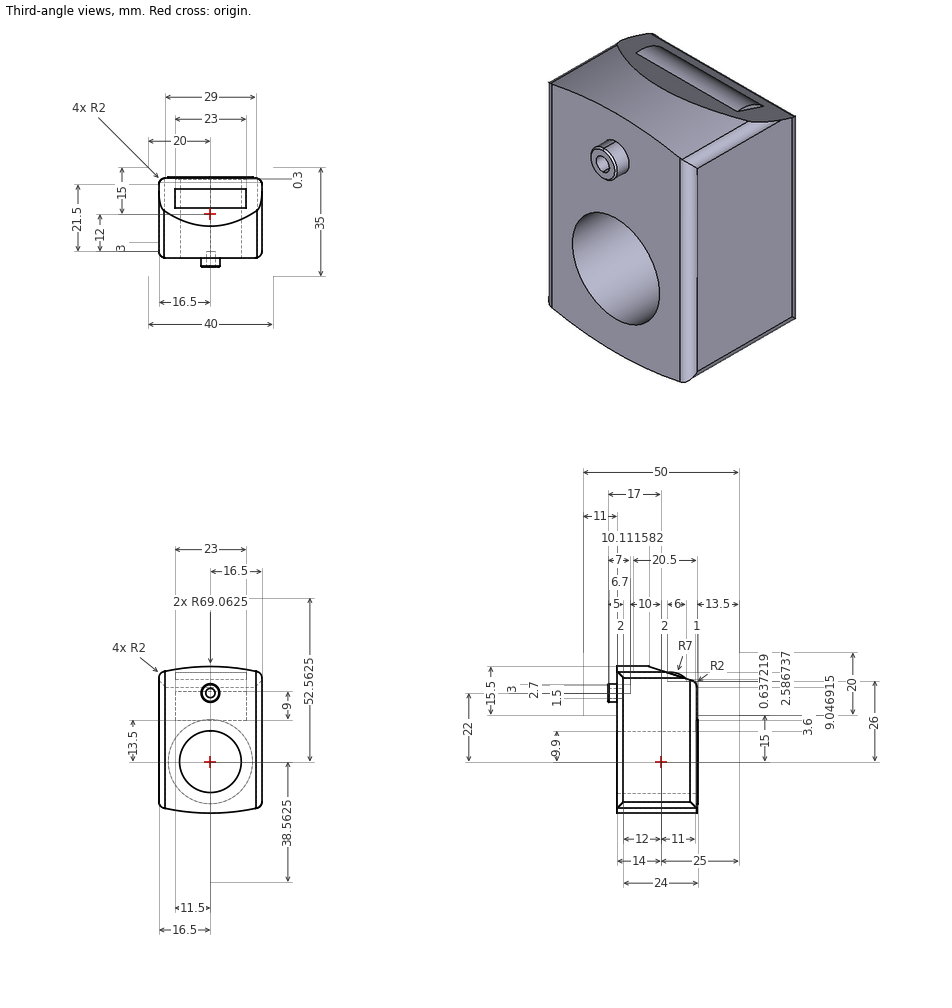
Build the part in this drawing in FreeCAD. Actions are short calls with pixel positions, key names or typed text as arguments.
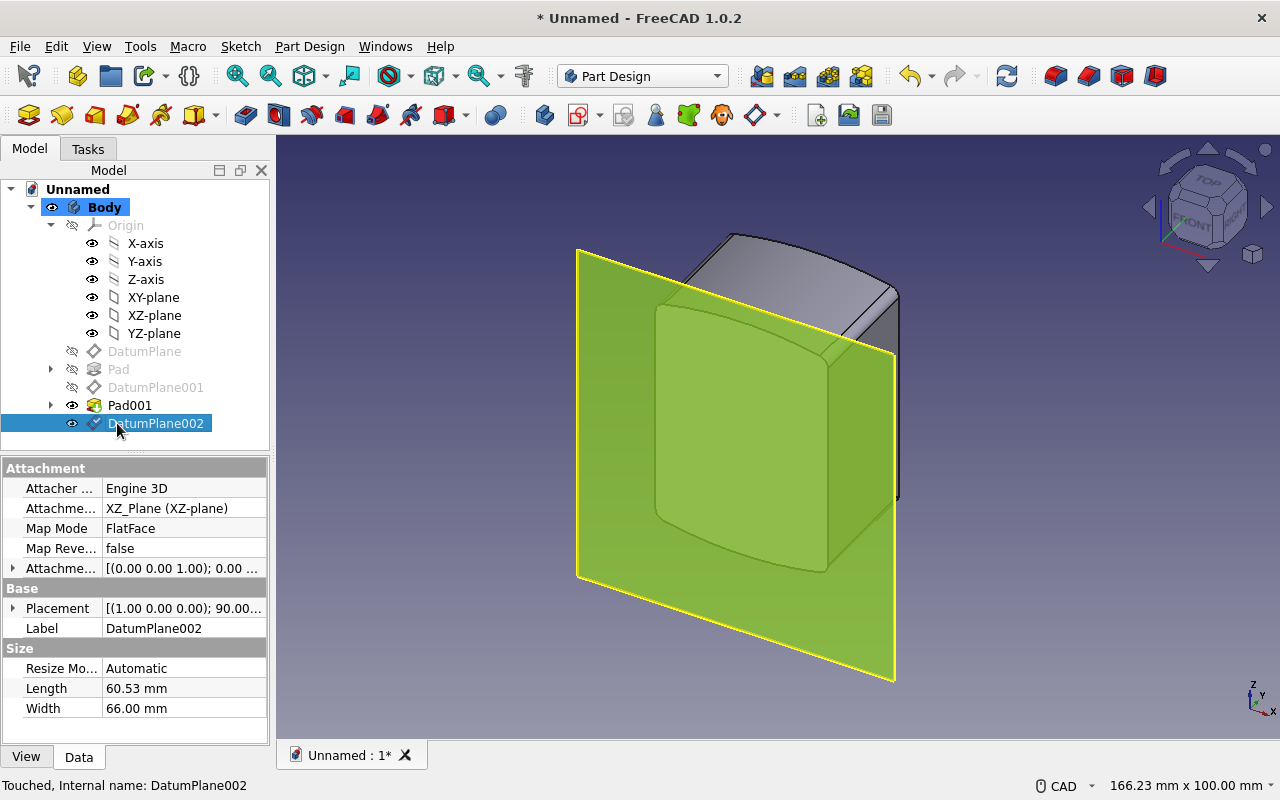
click(578, 116)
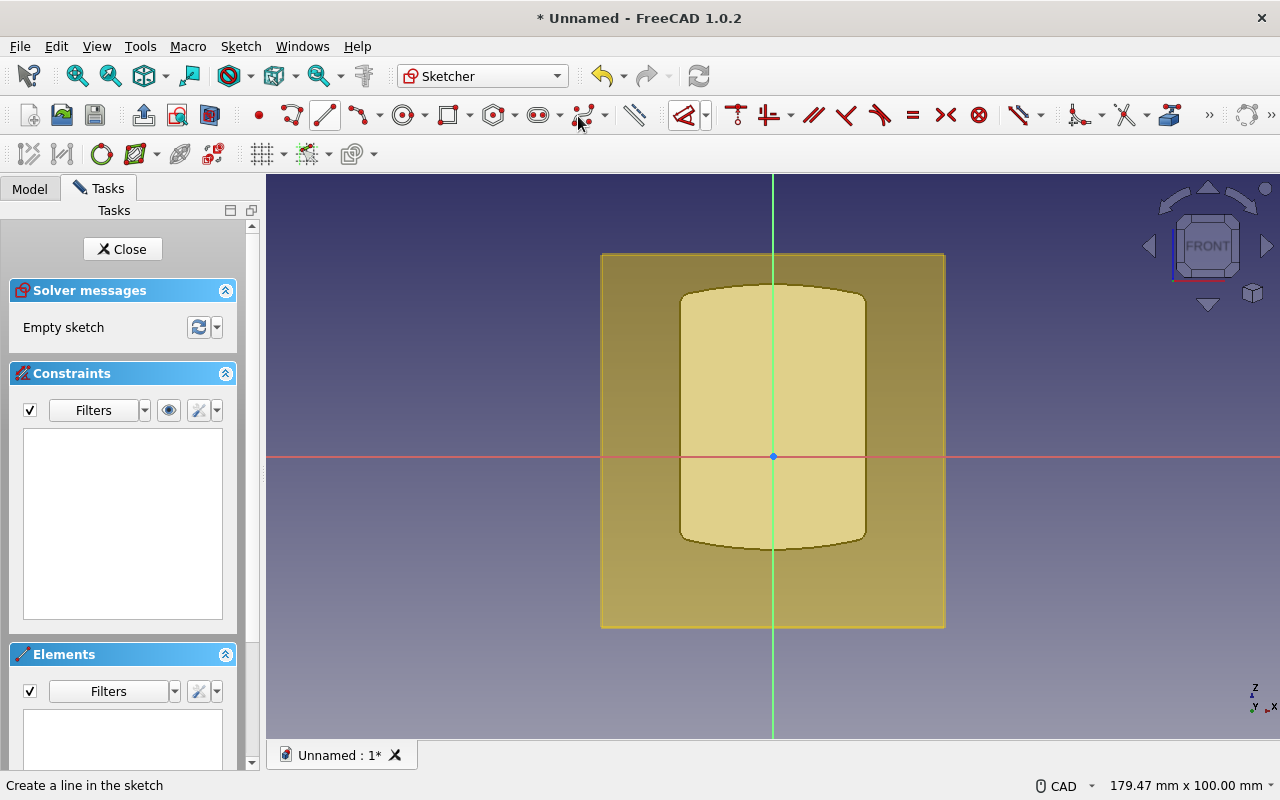
scroll(912, 337, up, 2)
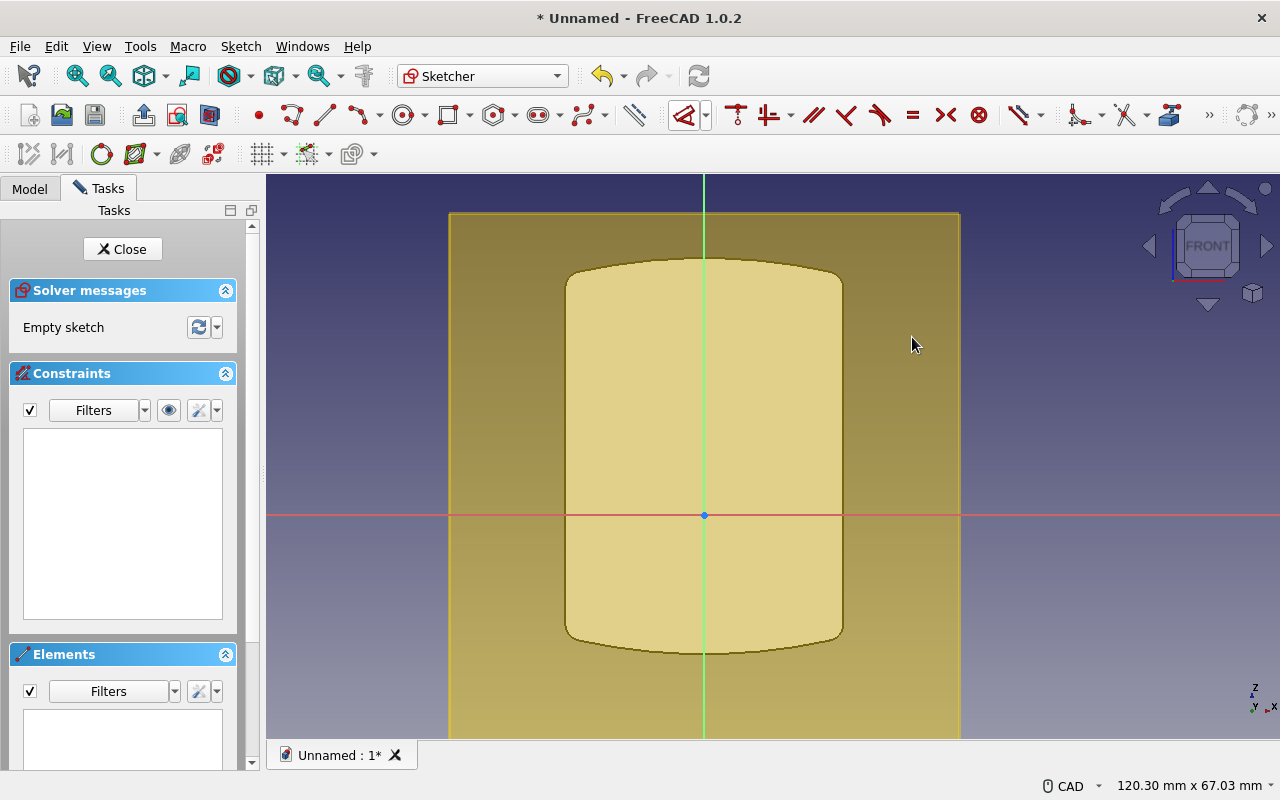
click(325, 116)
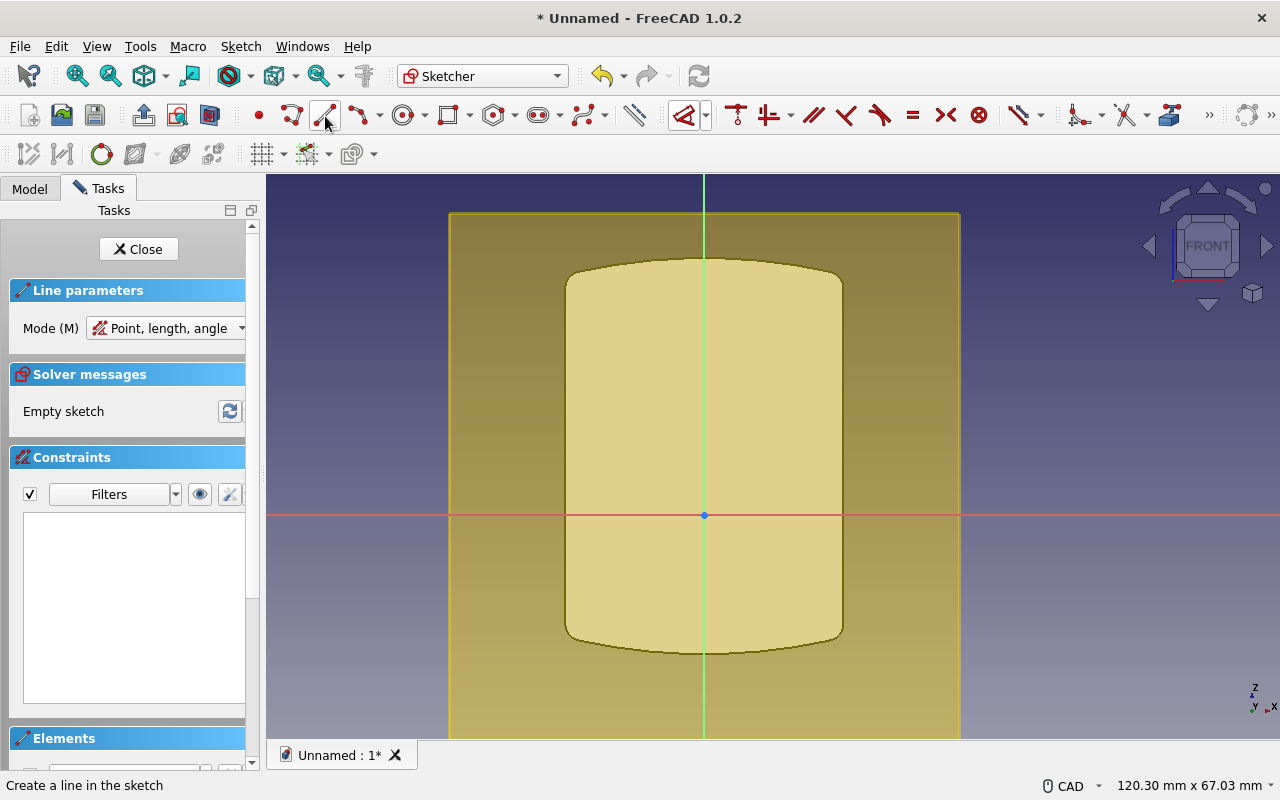
click(565, 624)
click(565, 288)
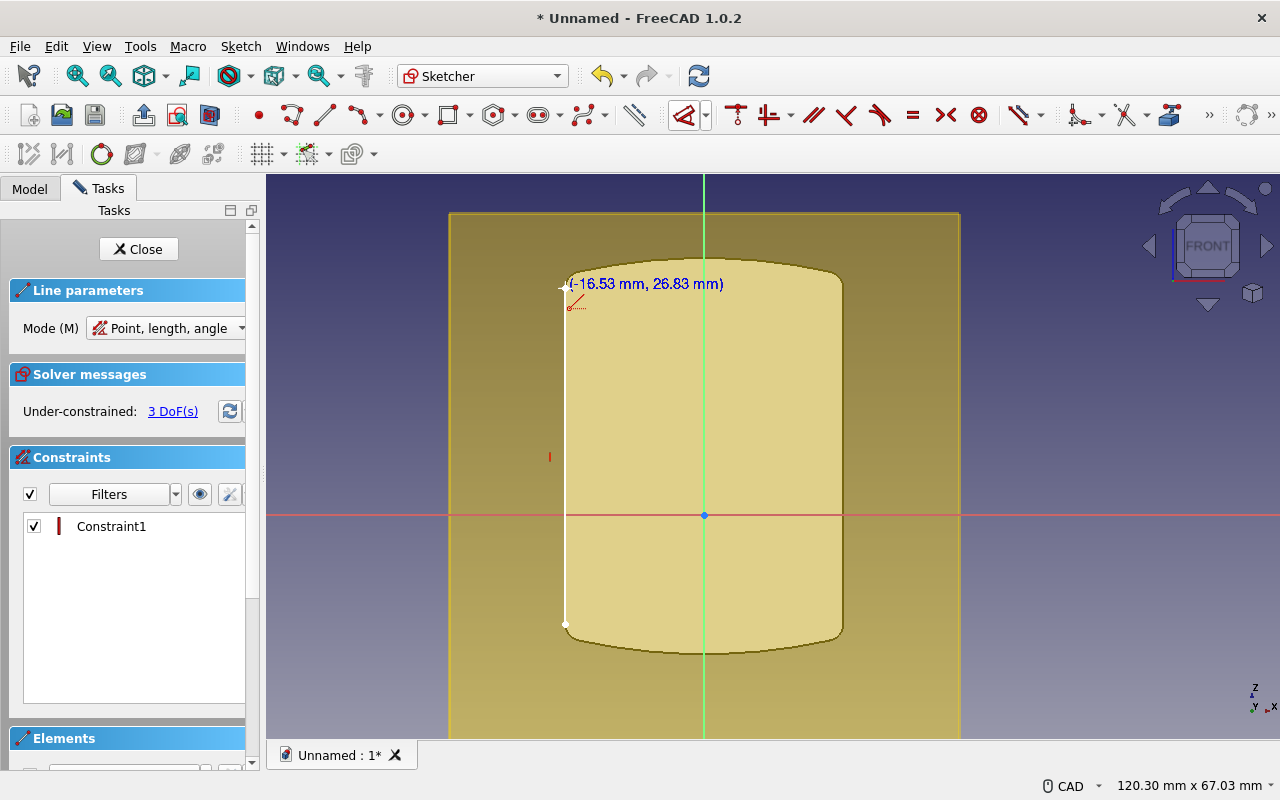
click(843, 288)
click(843, 624)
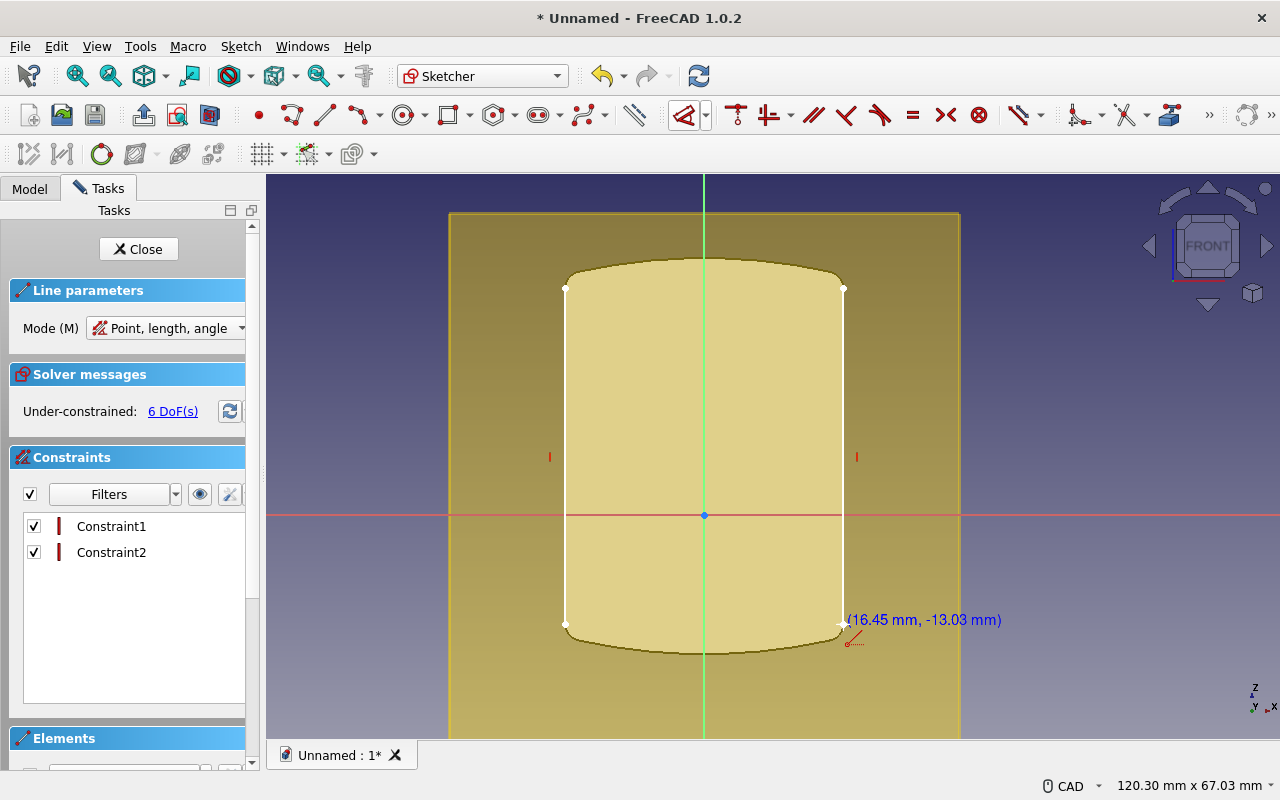
click(358, 116)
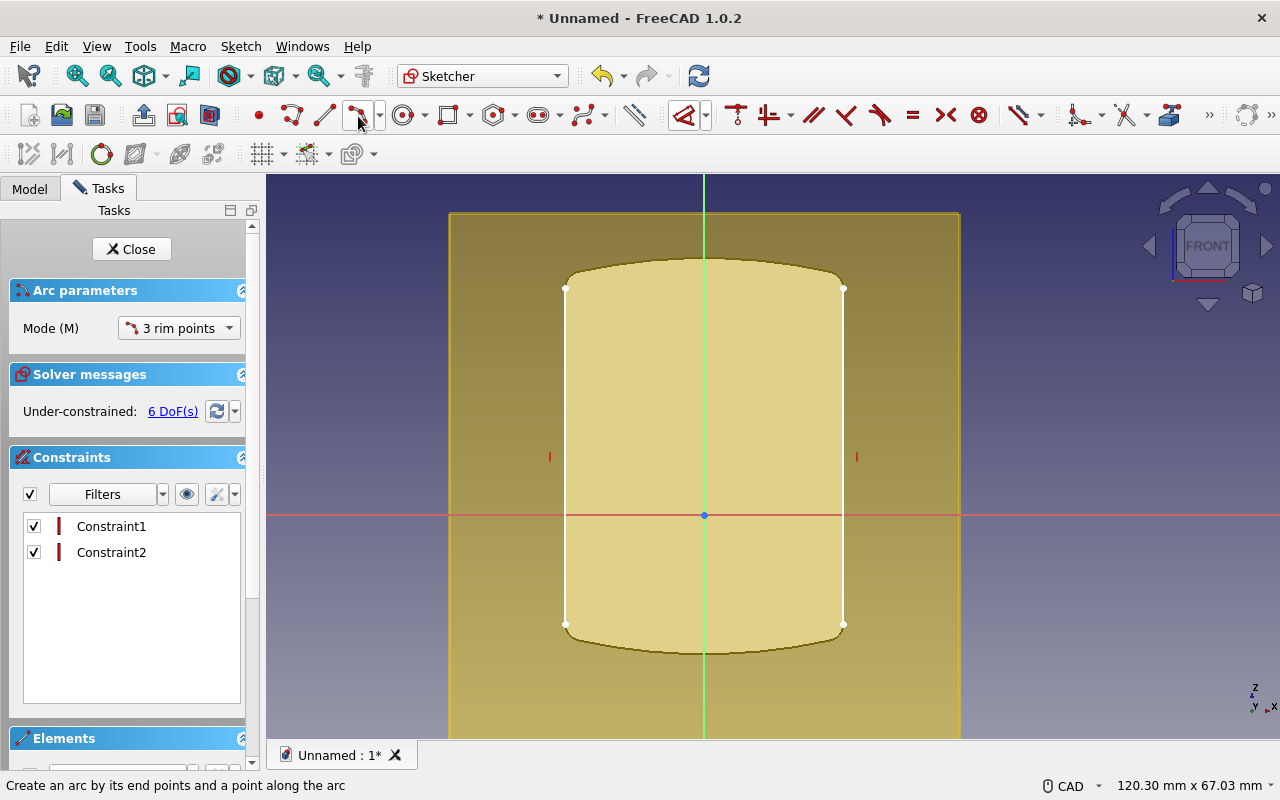
click(565, 289)
click(578, 272)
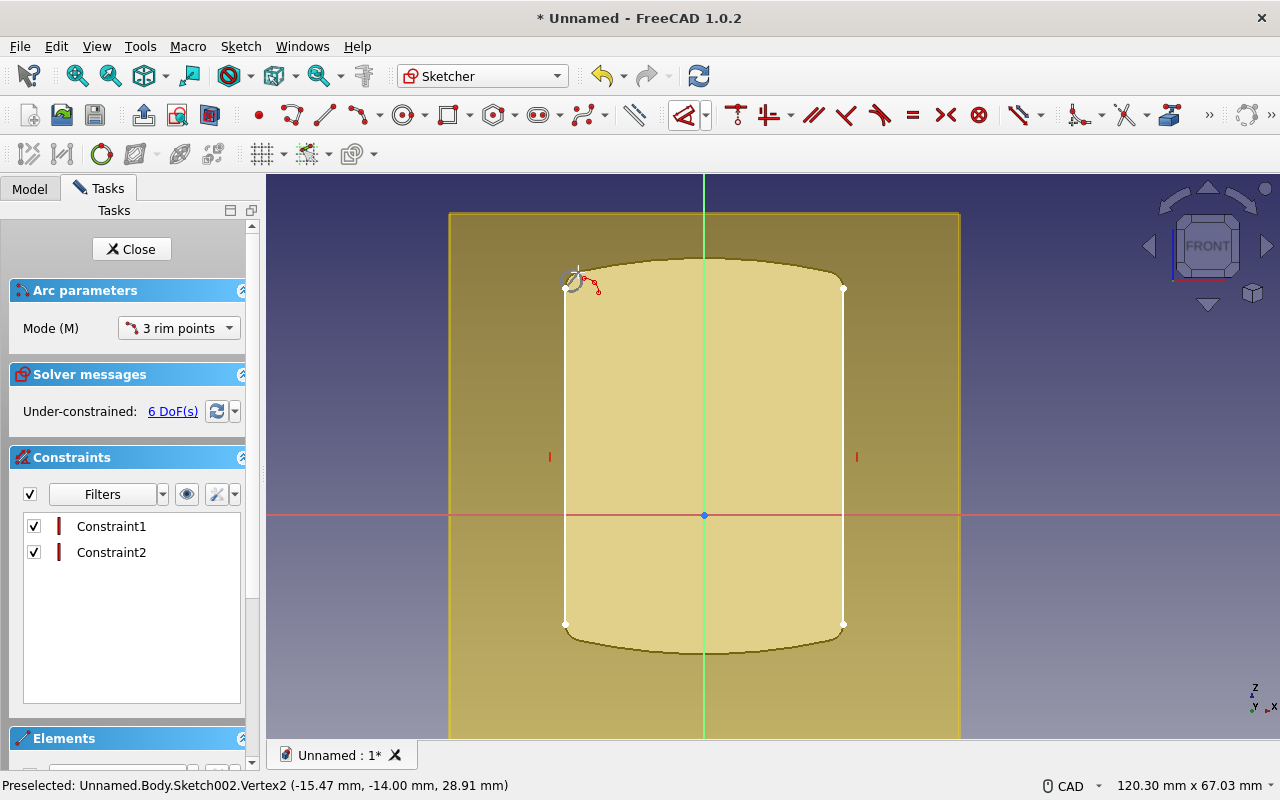
scroll(569, 278, up, 8)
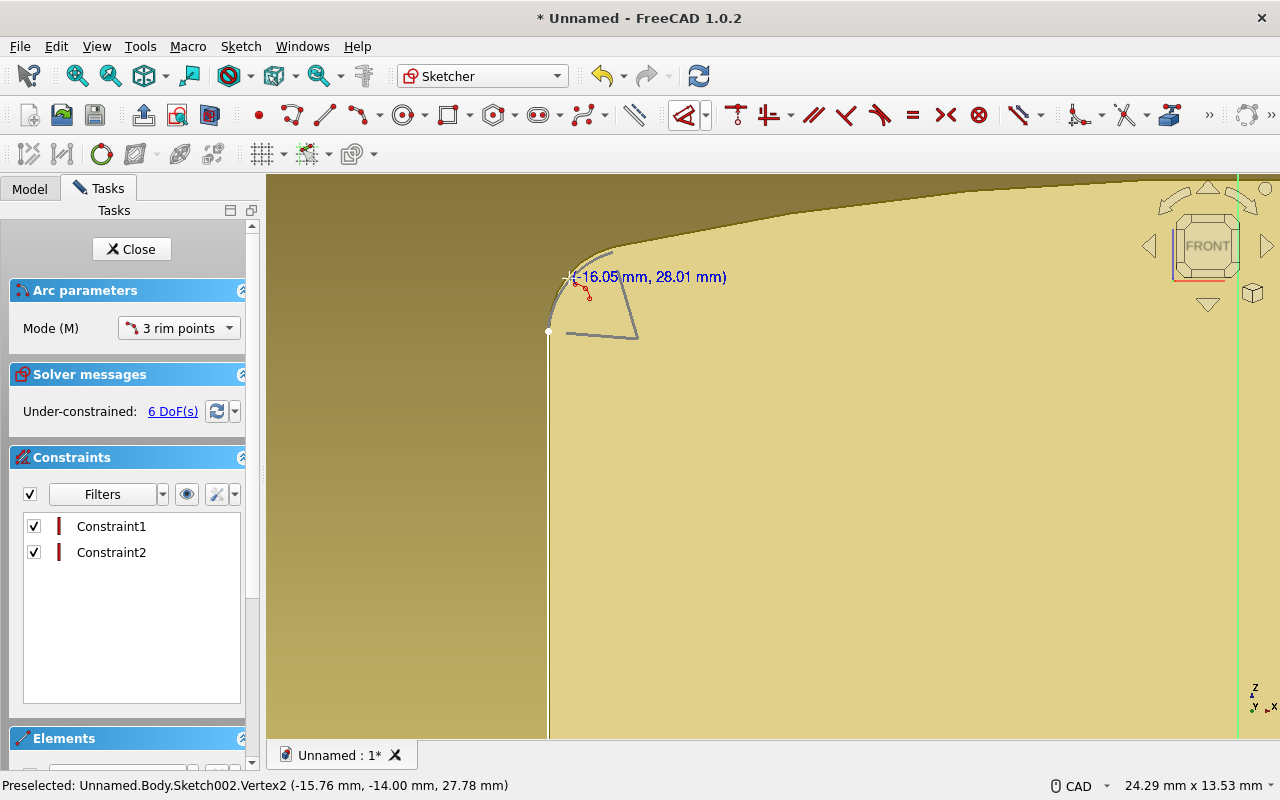
click(568, 276)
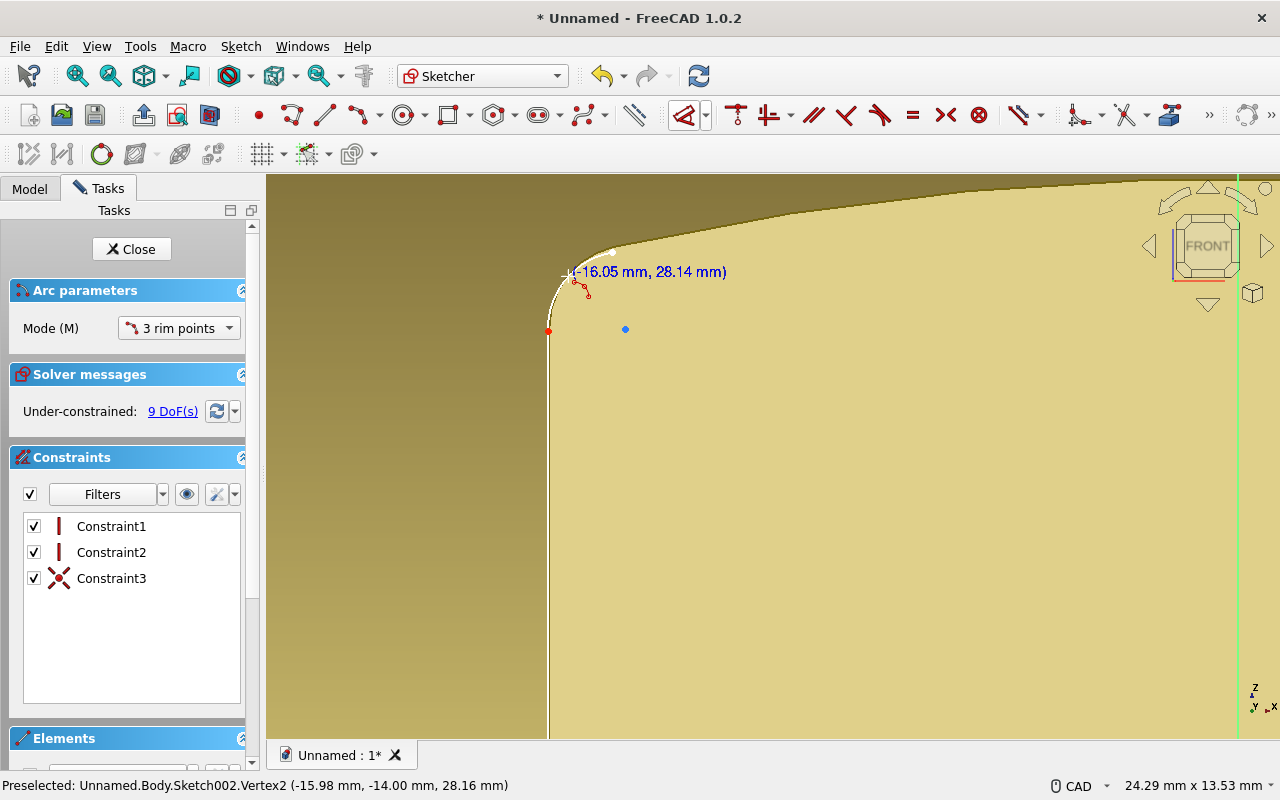
scroll(570, 279, down, 8)